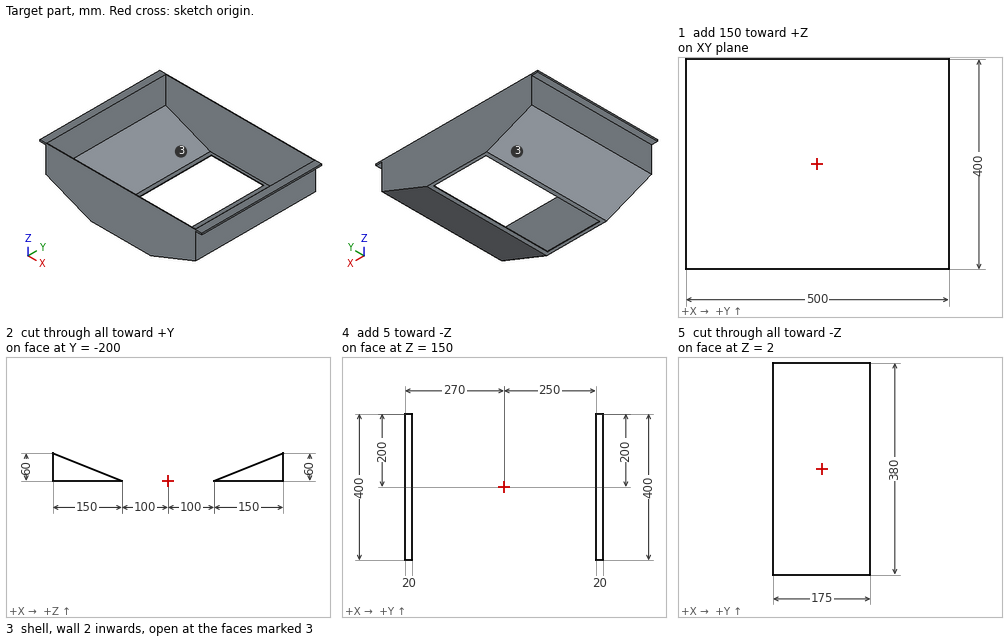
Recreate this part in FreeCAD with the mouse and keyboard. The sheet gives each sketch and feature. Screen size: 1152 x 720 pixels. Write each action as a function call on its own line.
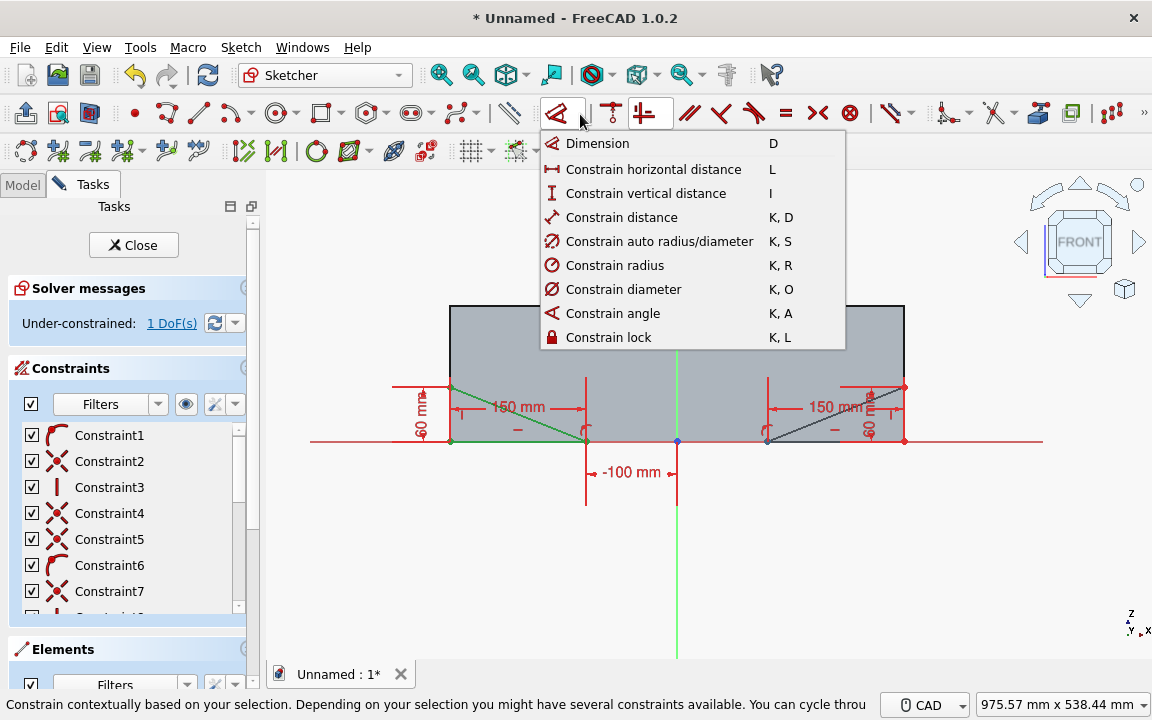
click(693, 169)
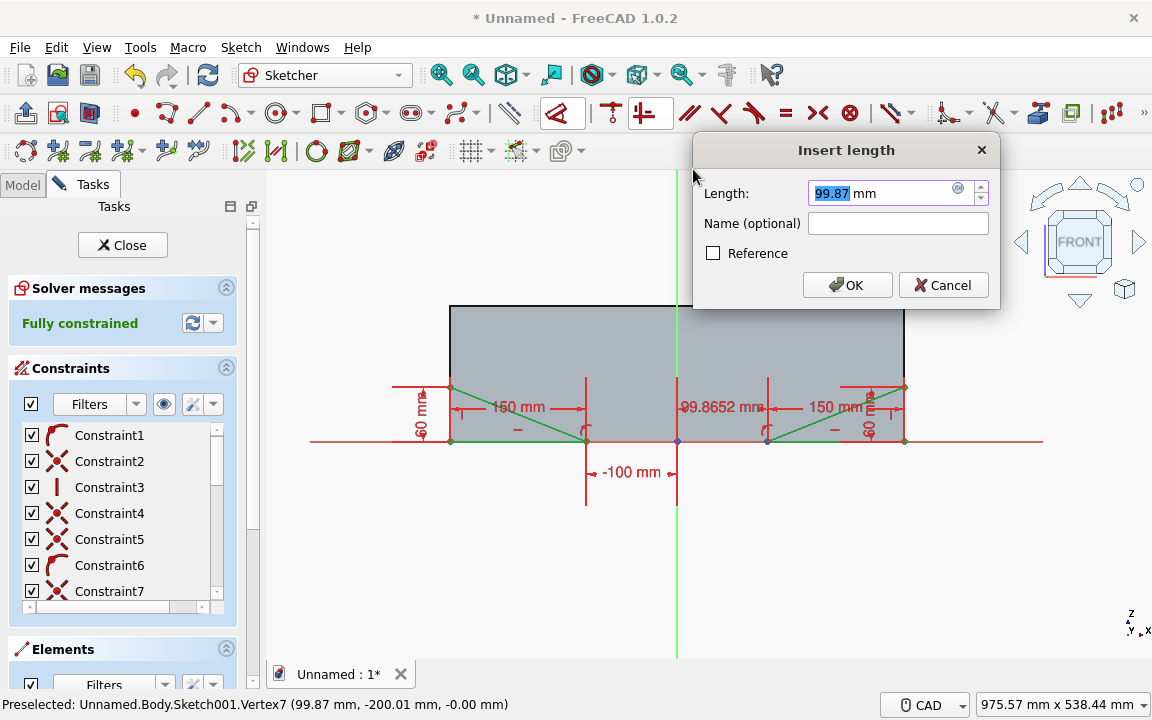
text(100)
key(Return)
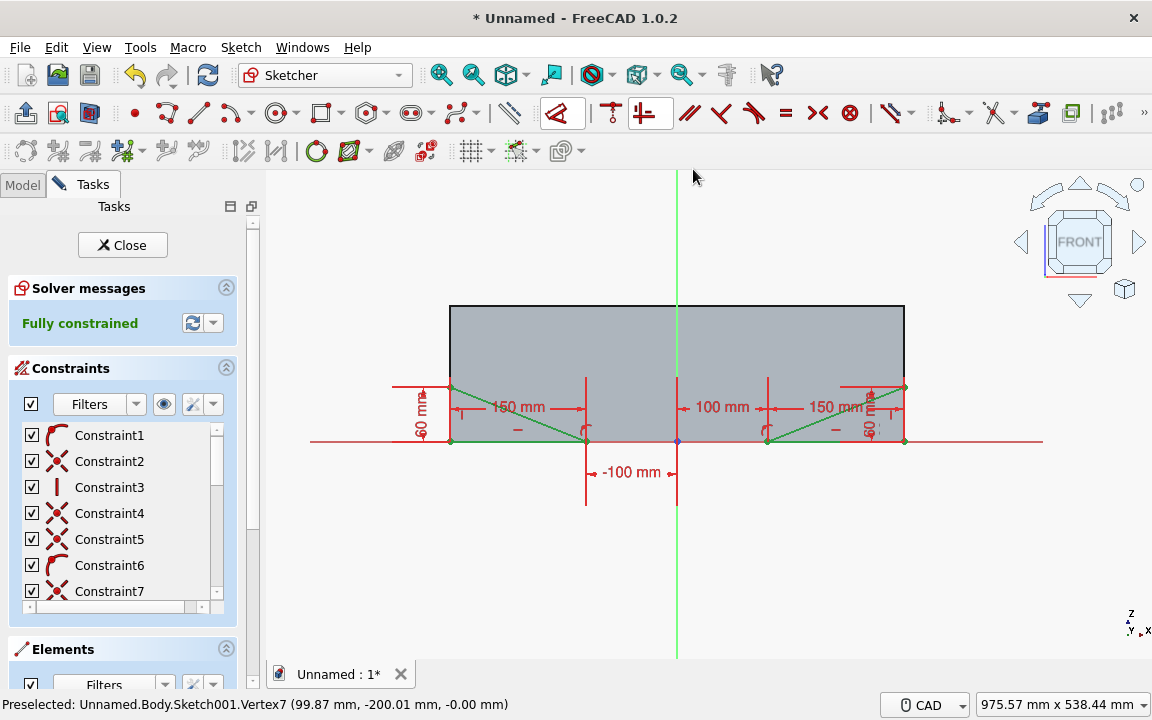
click(123, 245)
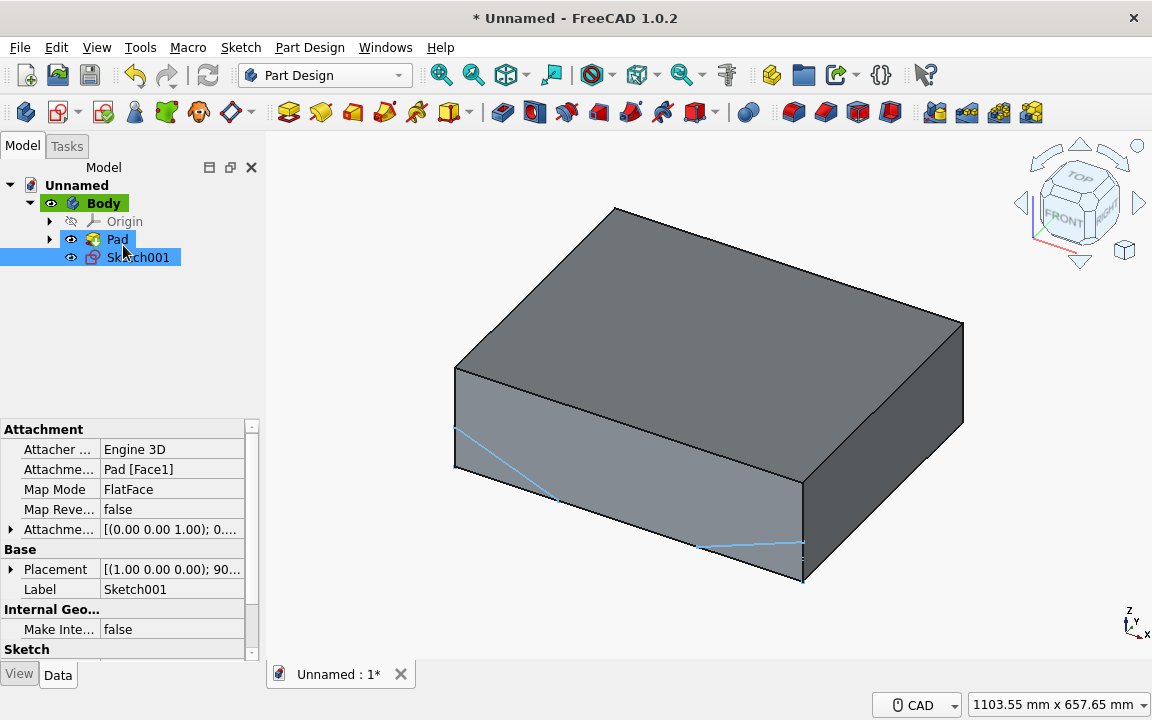
click(504, 112)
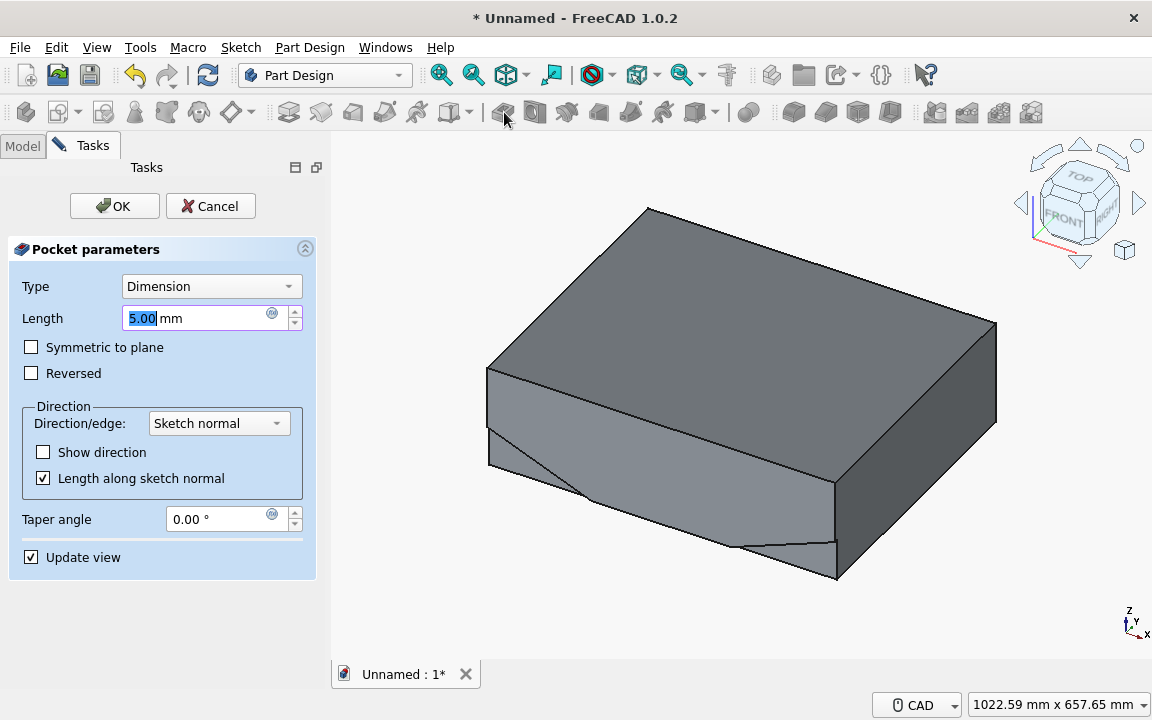
click(212, 286)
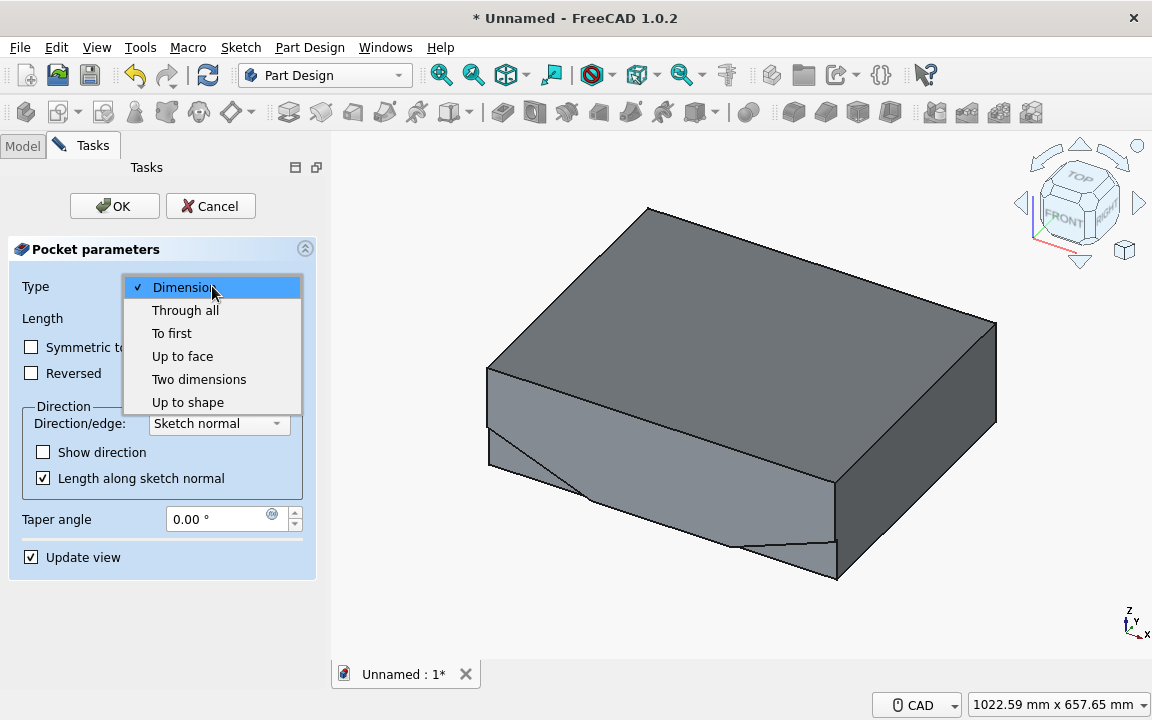
click(212, 310)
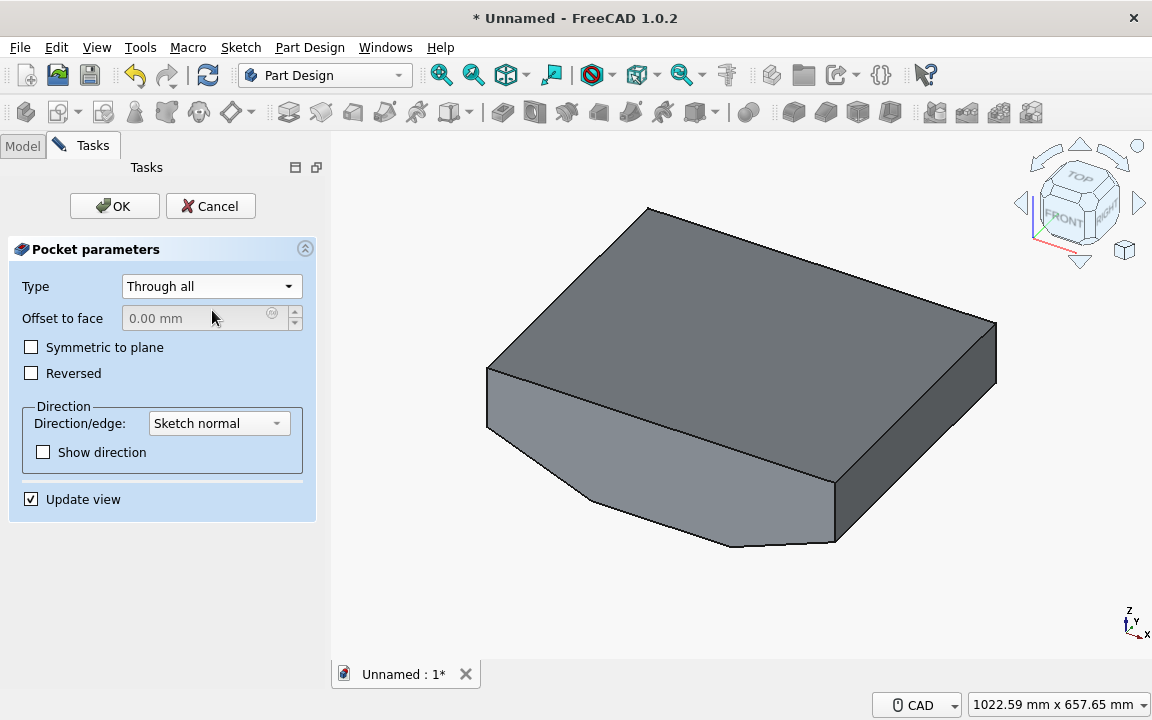
click(115, 206)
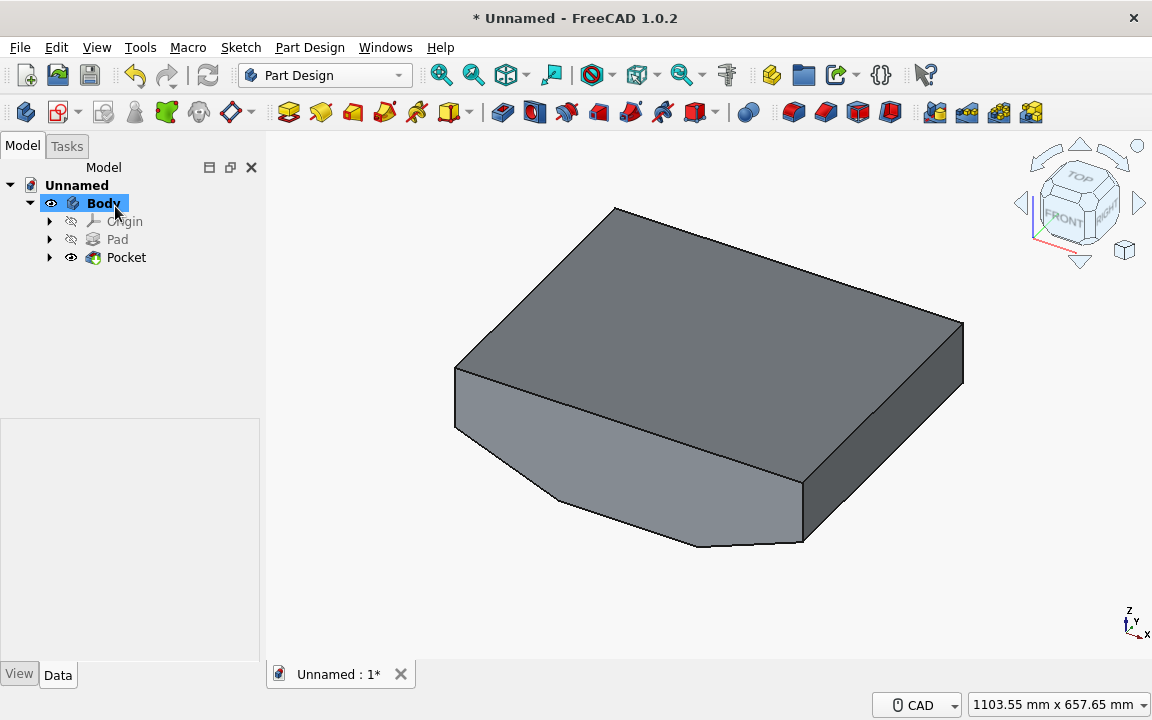
click(709, 345)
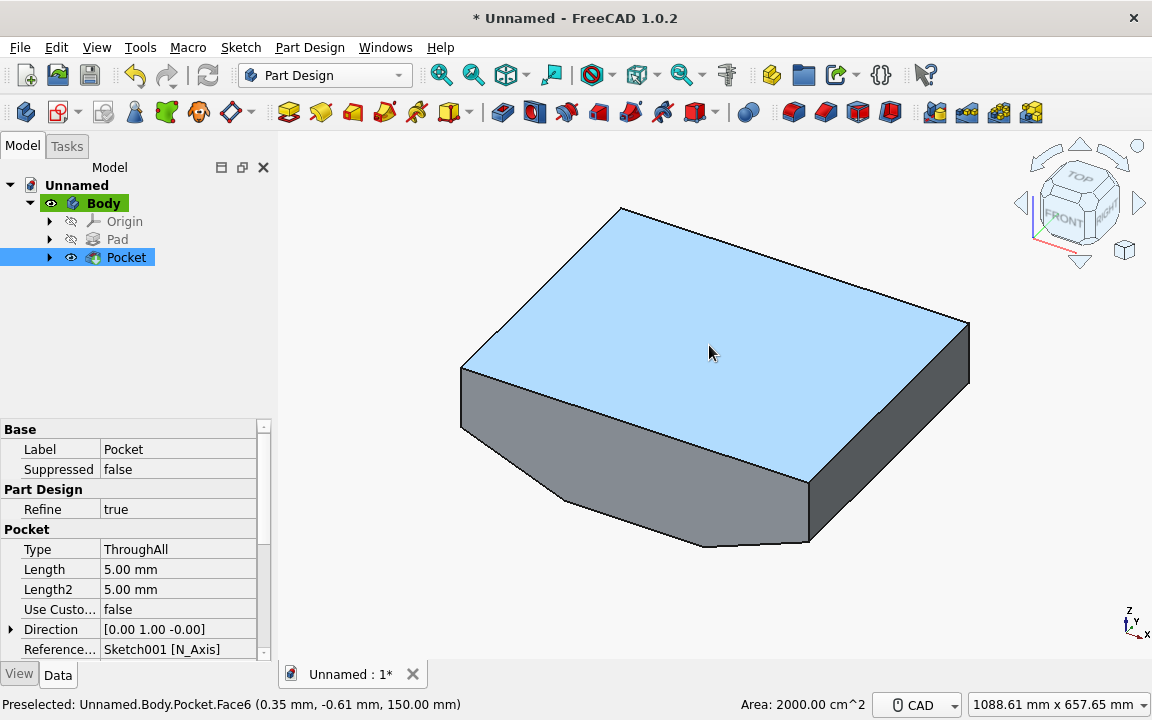
click(890, 112)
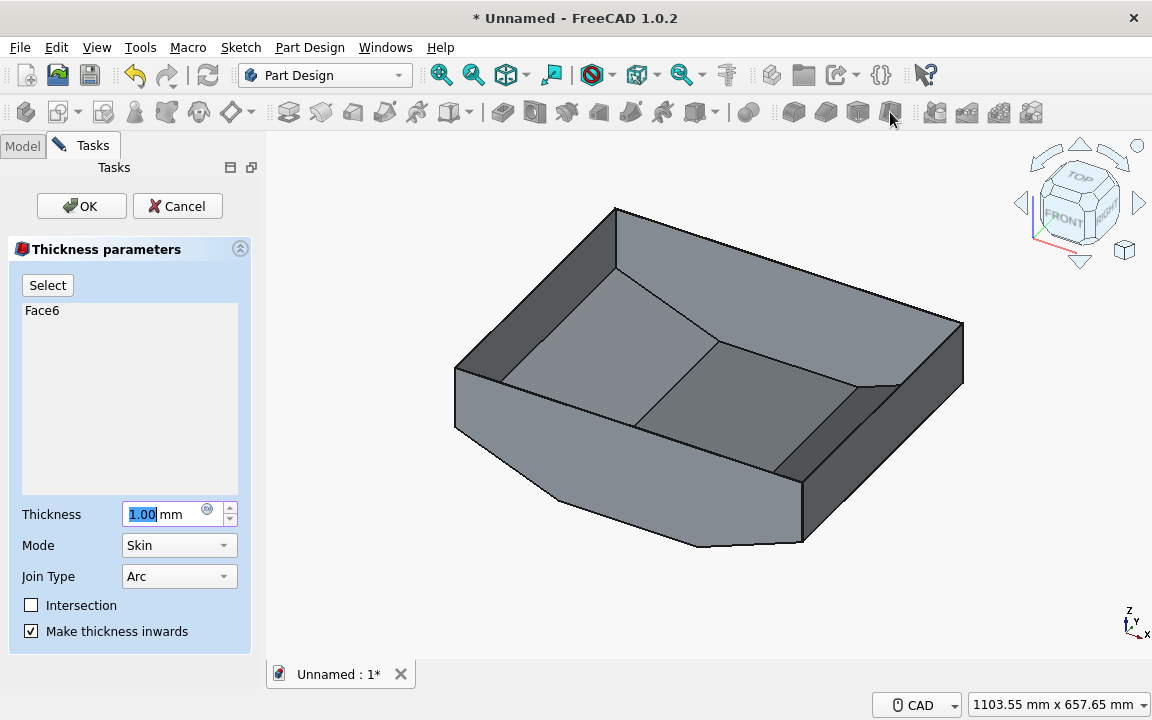
text(2)
key(Tab)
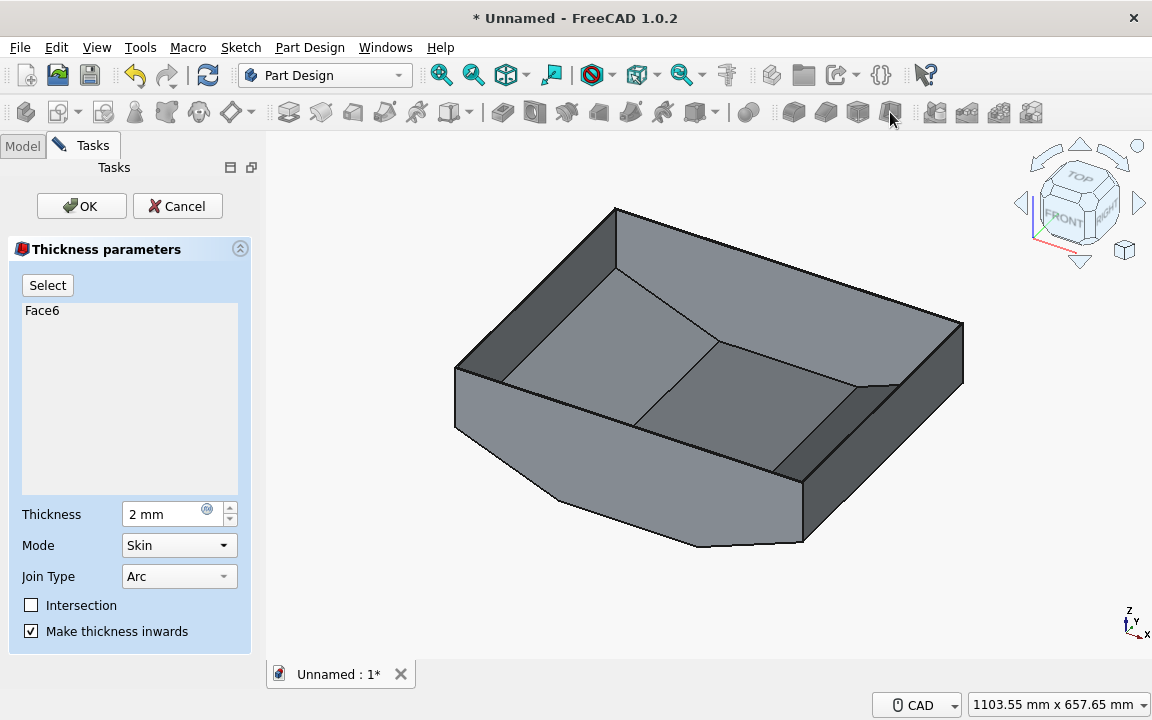
click(180, 576)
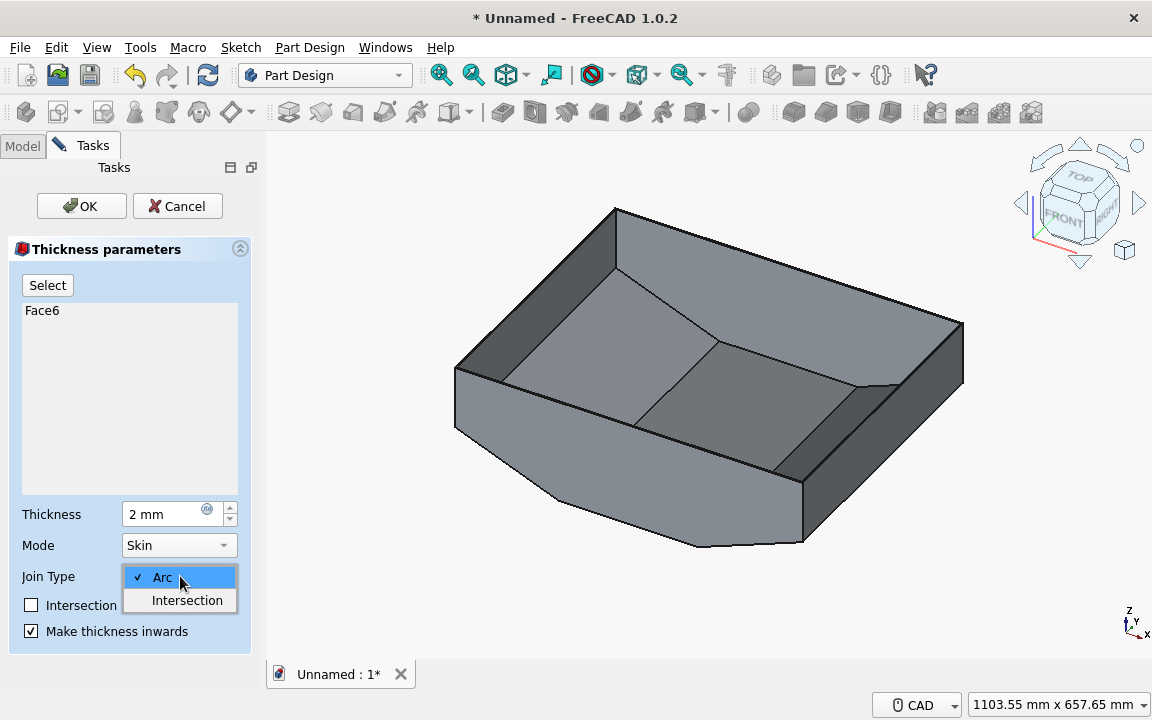
click(179, 600)